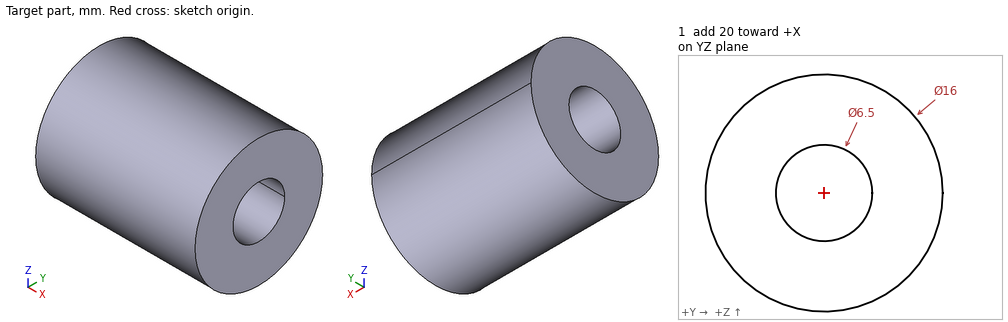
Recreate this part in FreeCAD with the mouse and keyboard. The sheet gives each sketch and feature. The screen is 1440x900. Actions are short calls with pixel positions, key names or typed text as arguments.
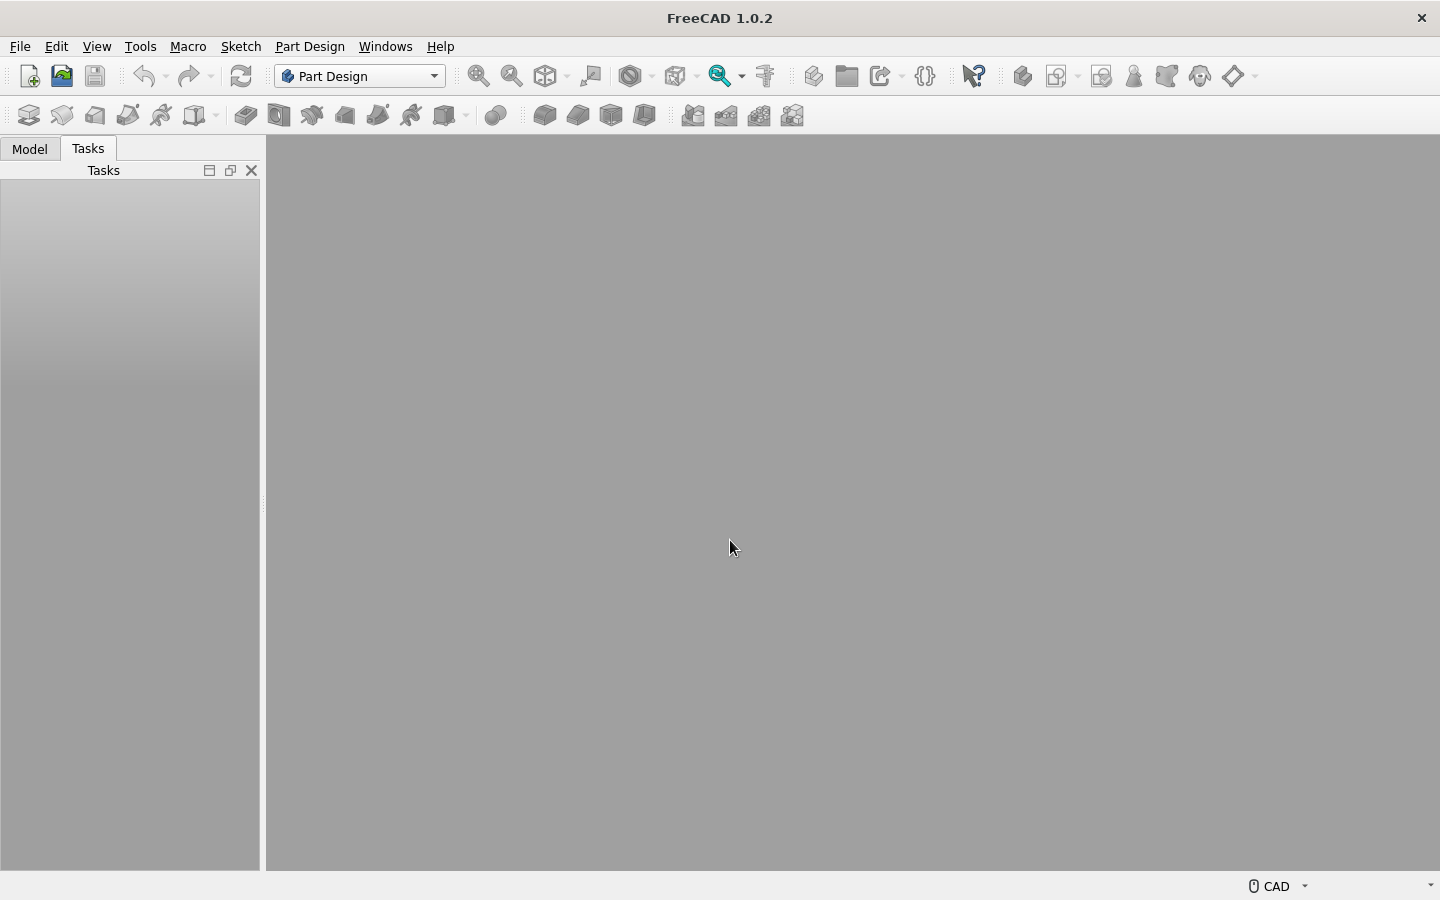
click(29, 76)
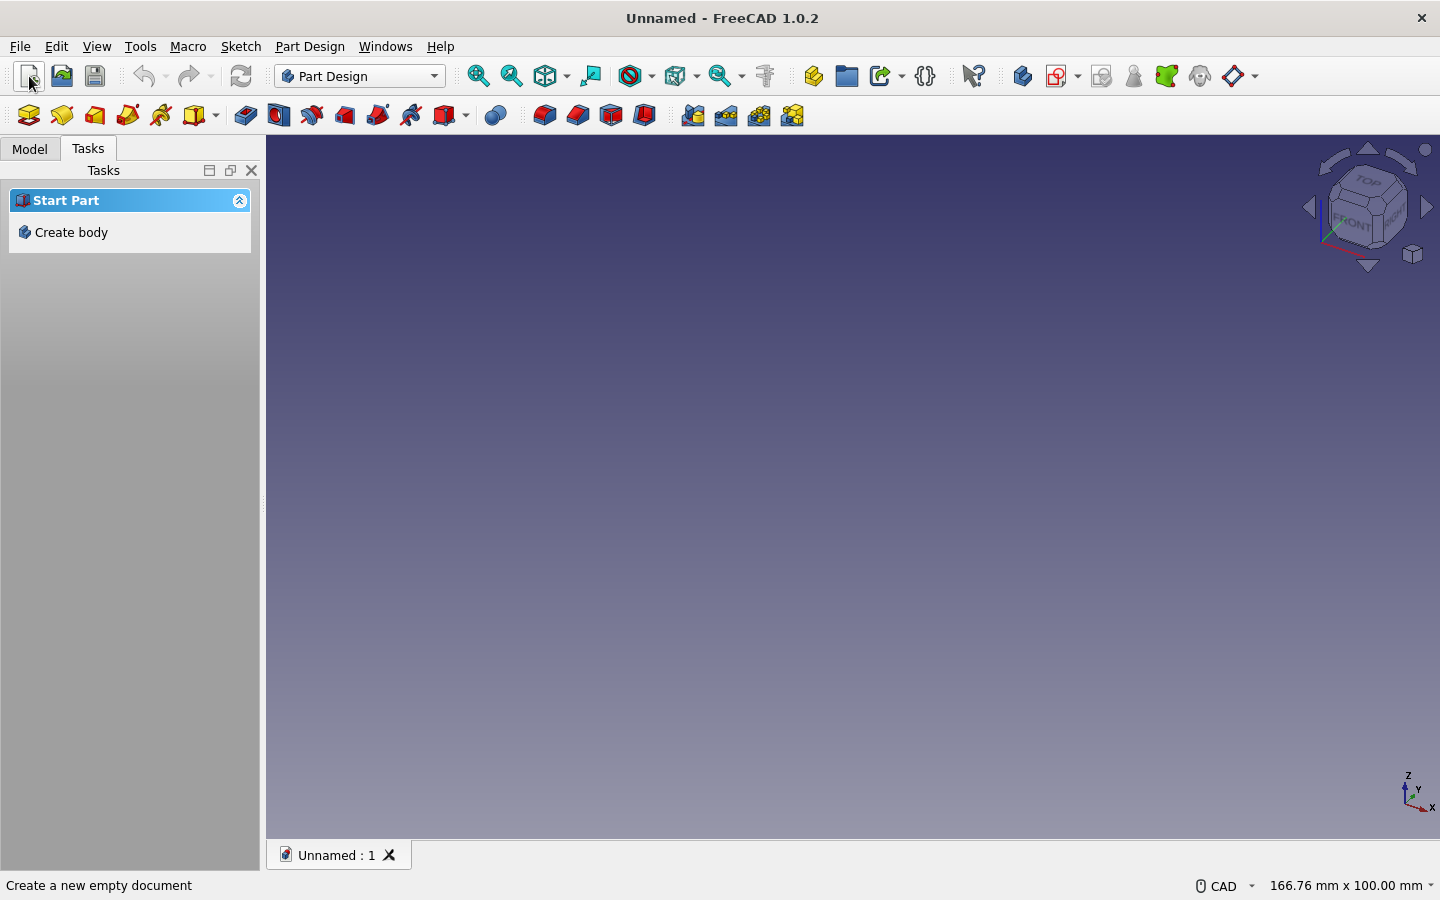
click(1056, 76)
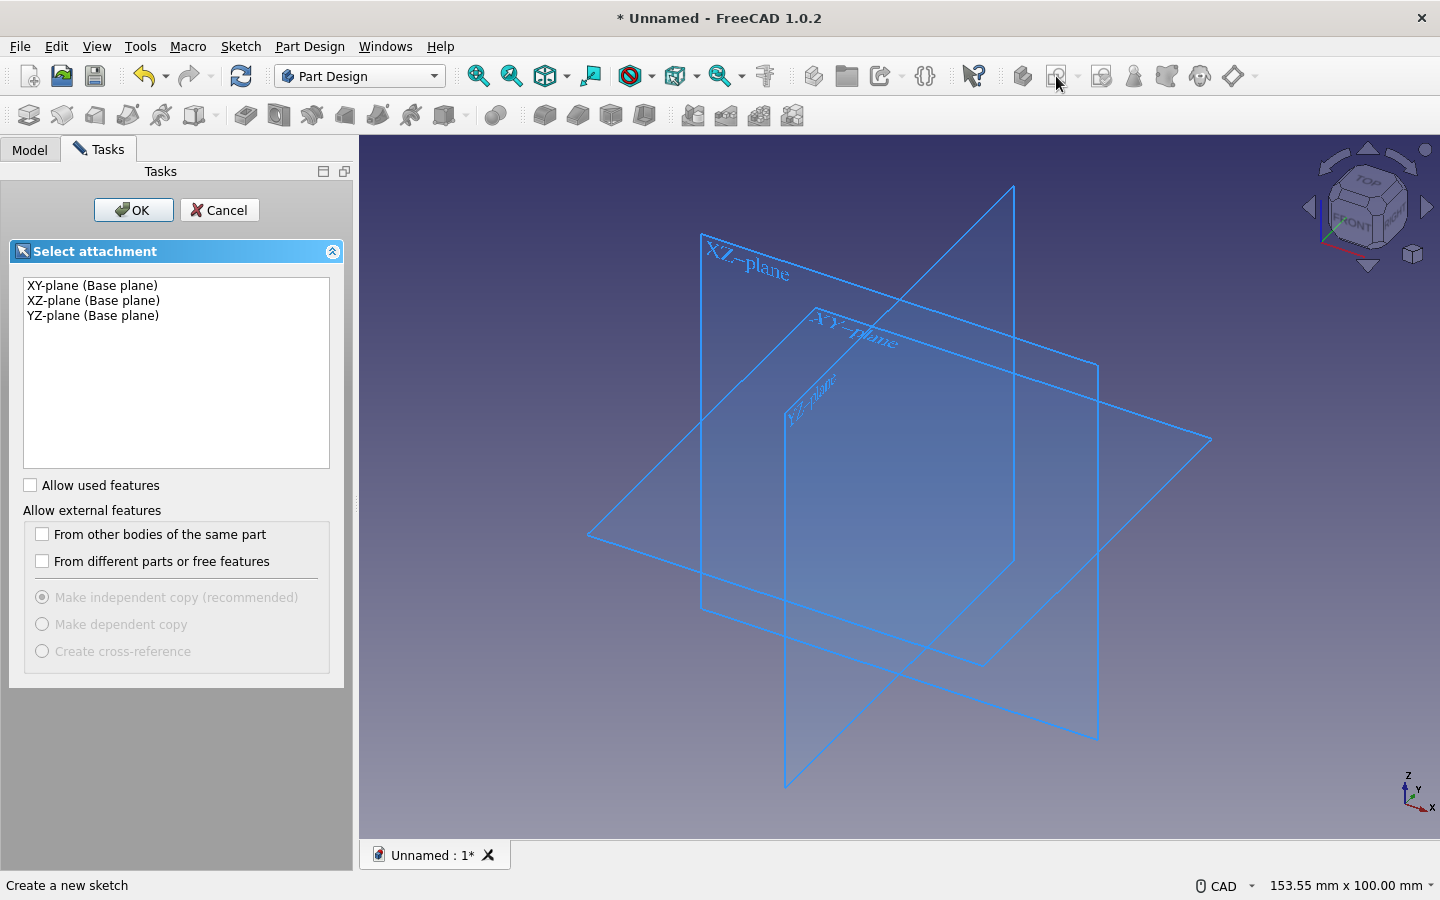
click(84, 316)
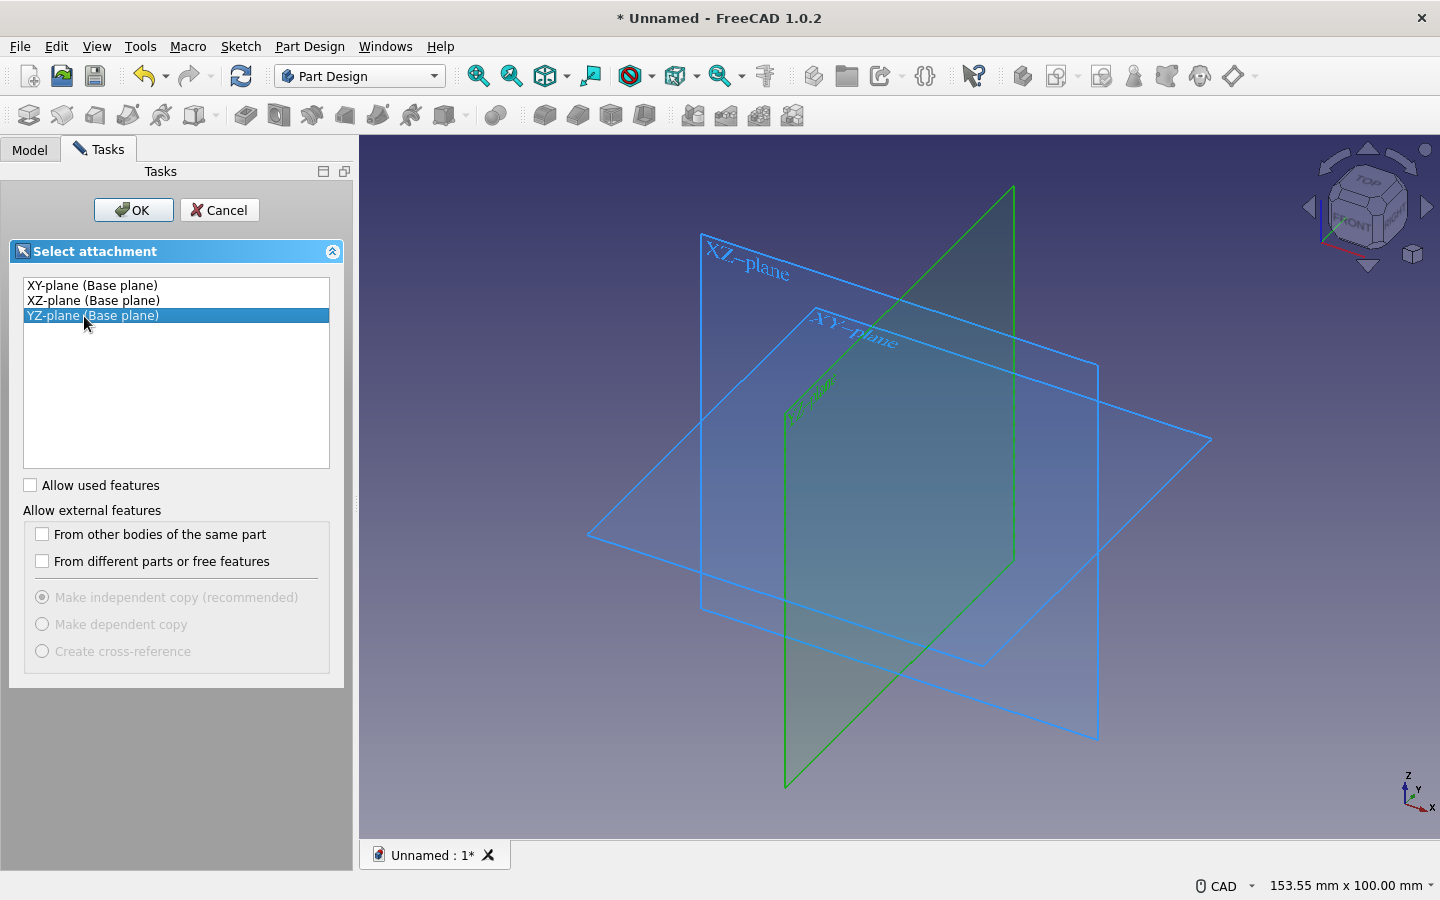
click(134, 210)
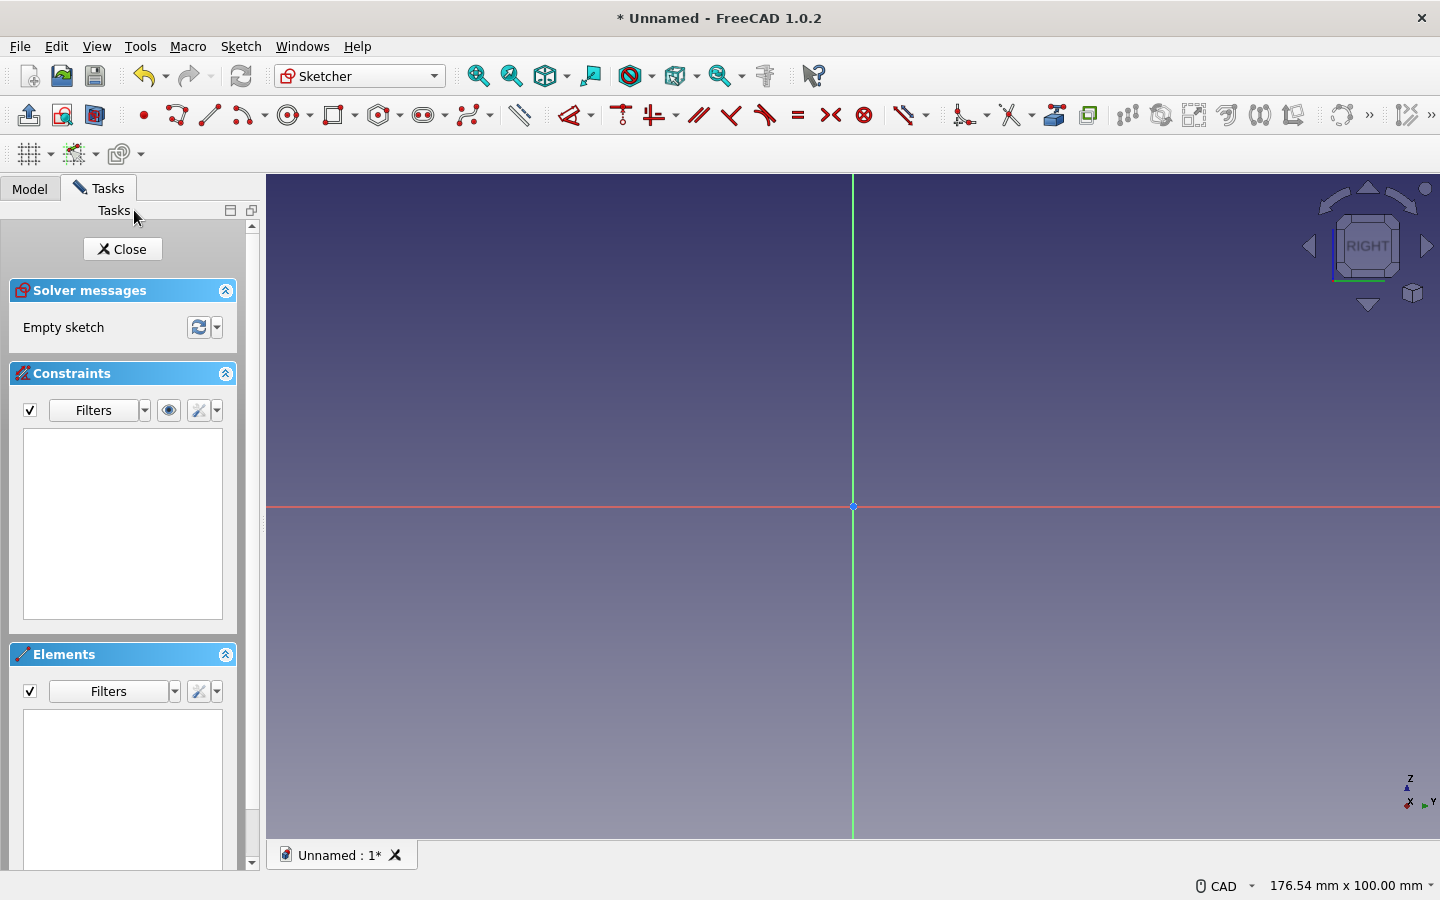
scroll(875, 507, up, 7)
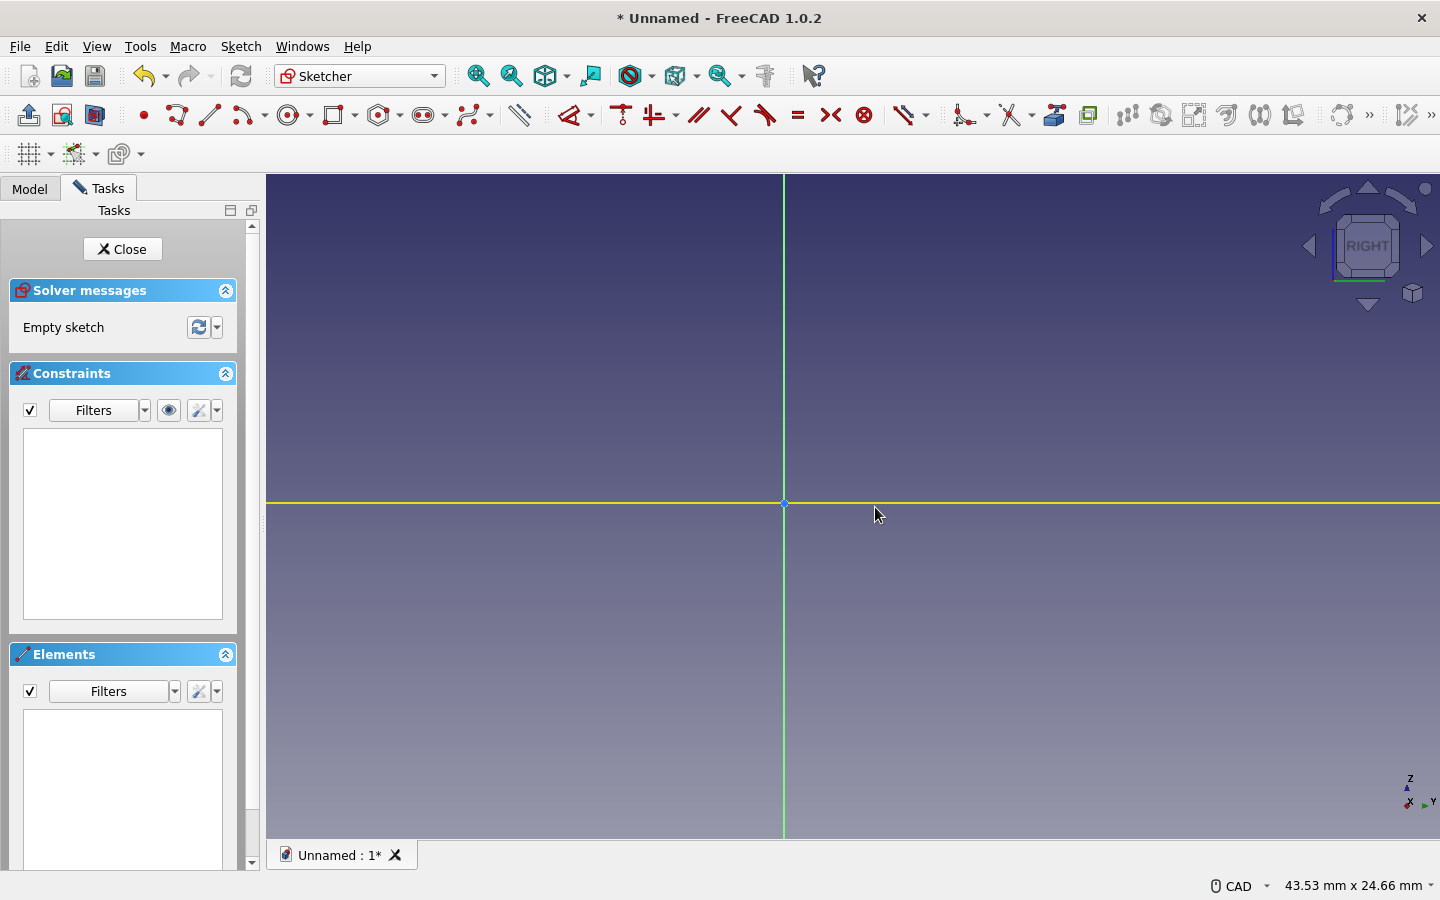
click(288, 116)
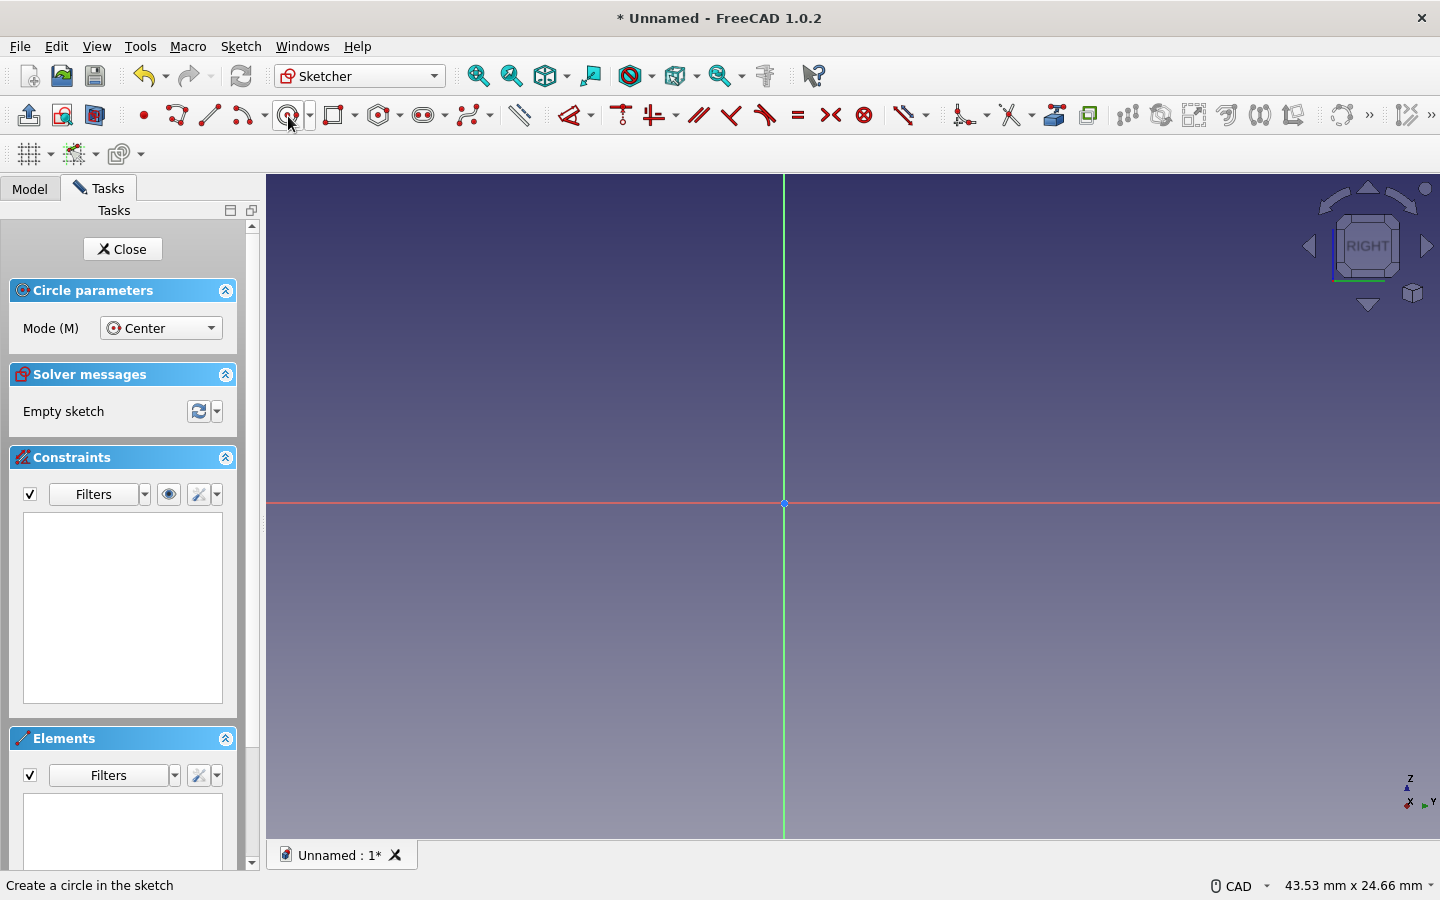
click(784, 503)
move(937, 351)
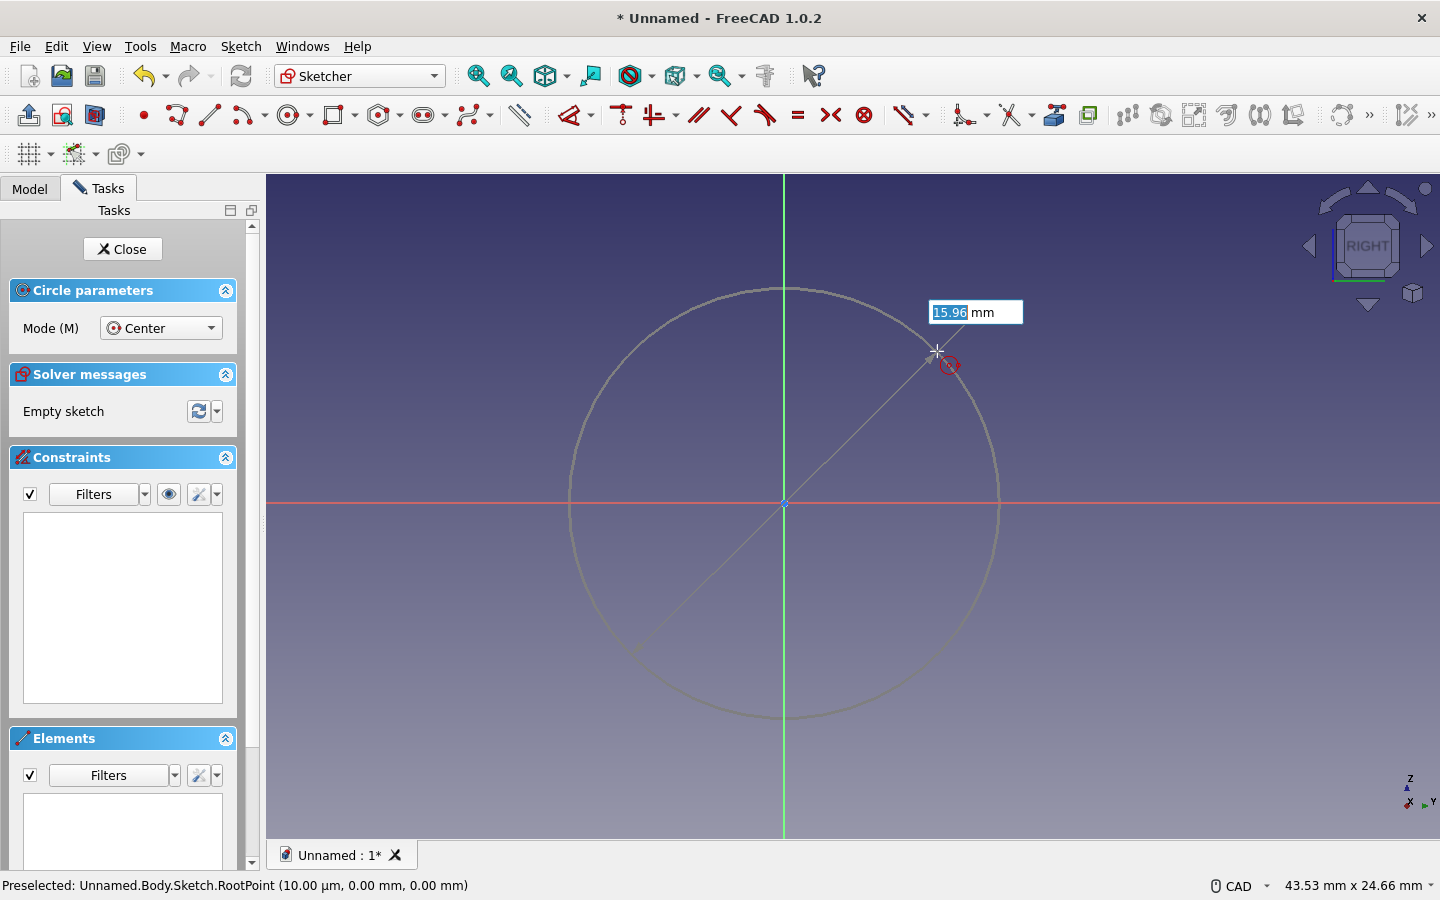
text(16)
key(Return)